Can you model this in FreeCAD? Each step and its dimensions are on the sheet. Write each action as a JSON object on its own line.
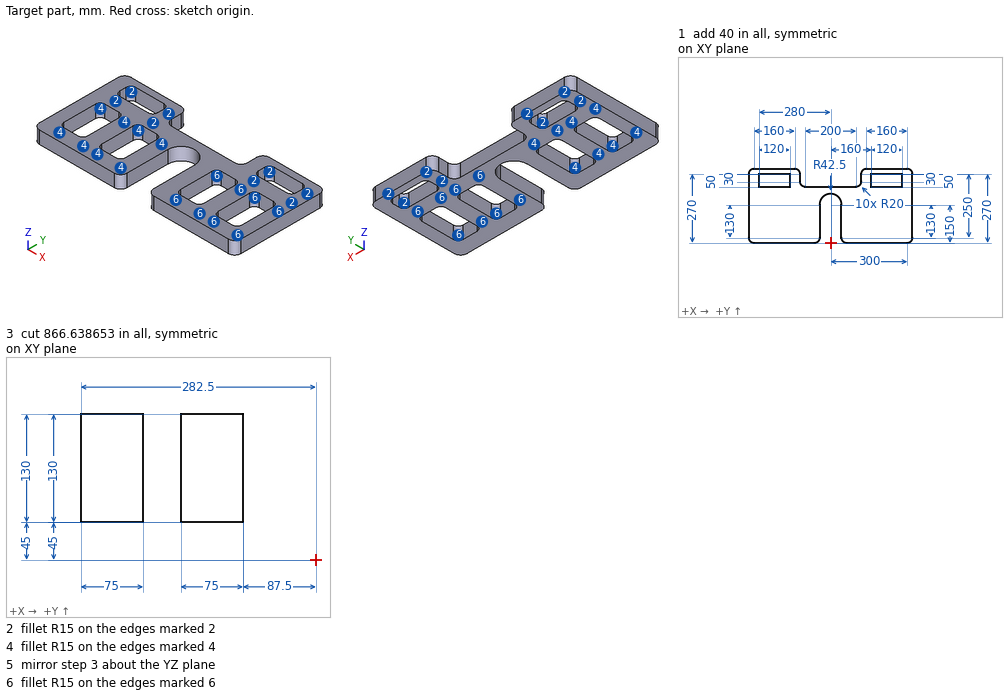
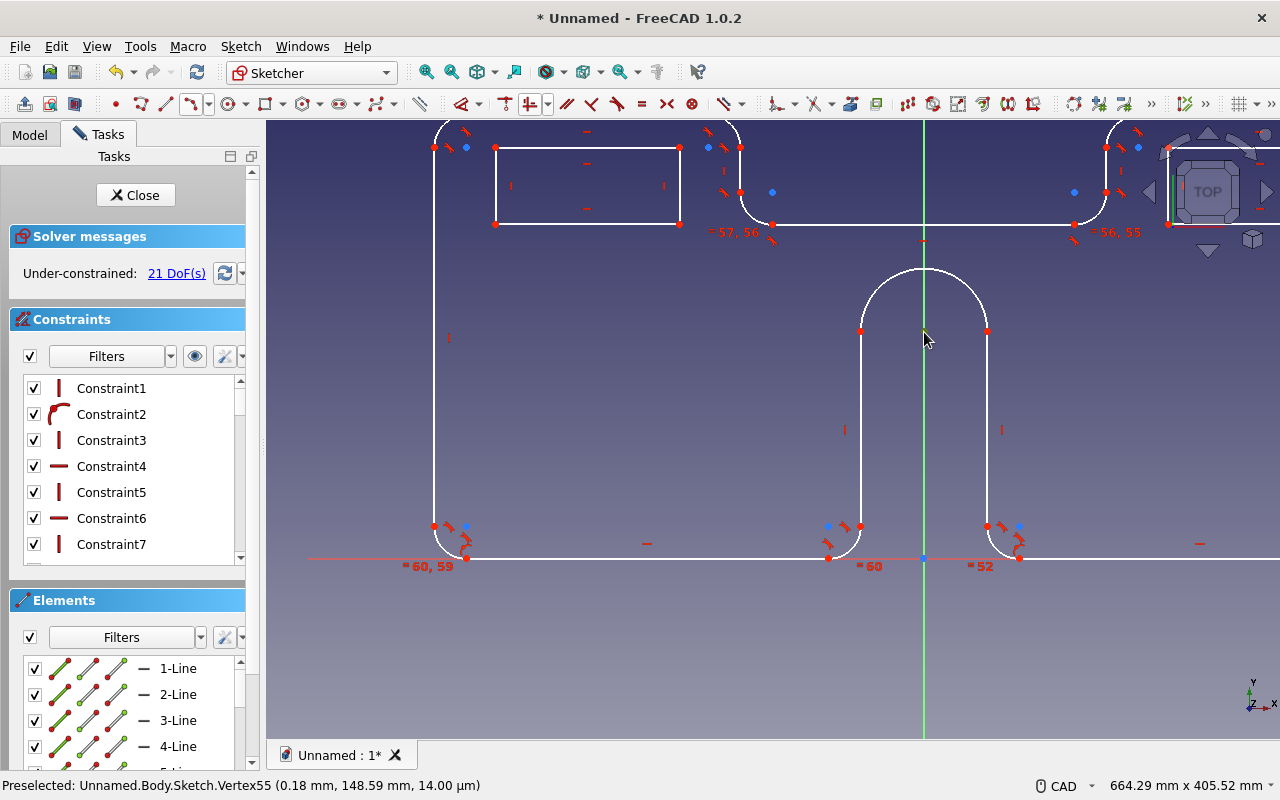
{"action": "left_click", "coordinate": [924, 671]}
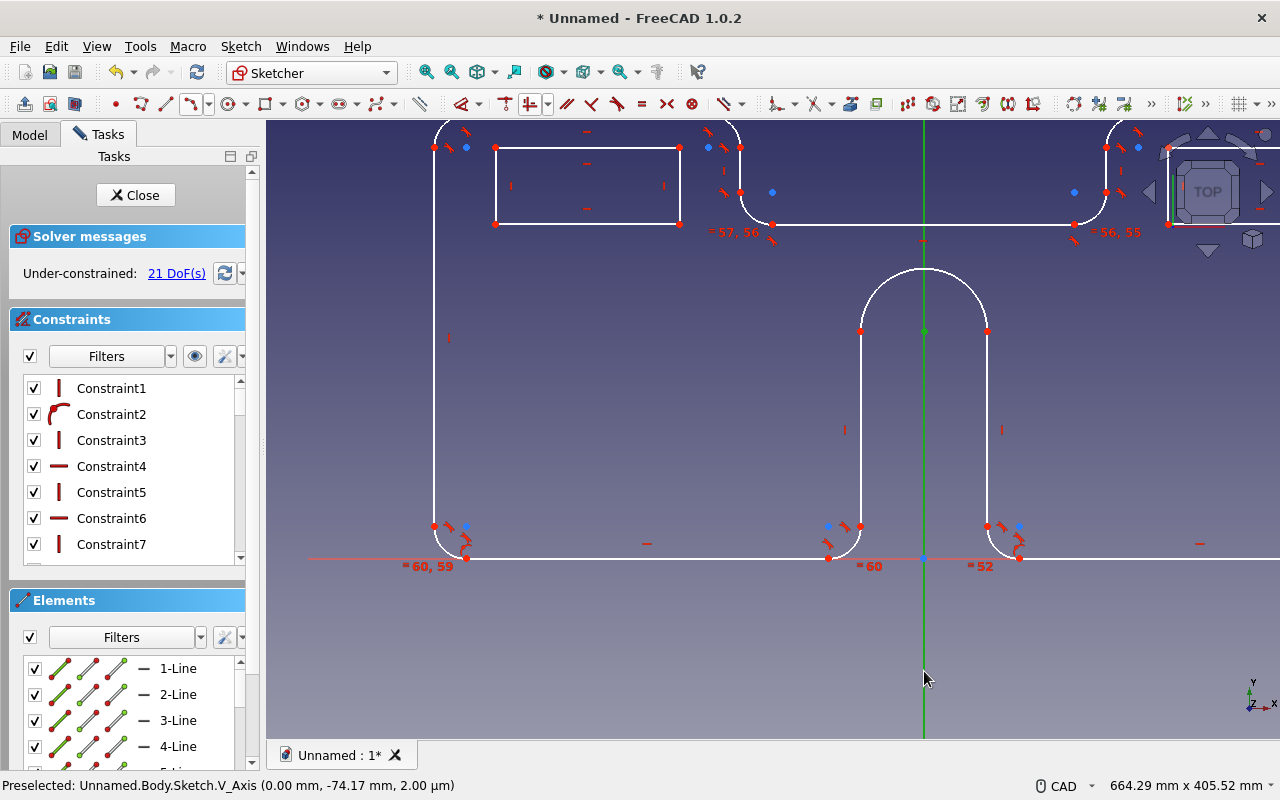
{"action": "key", "text": "c"}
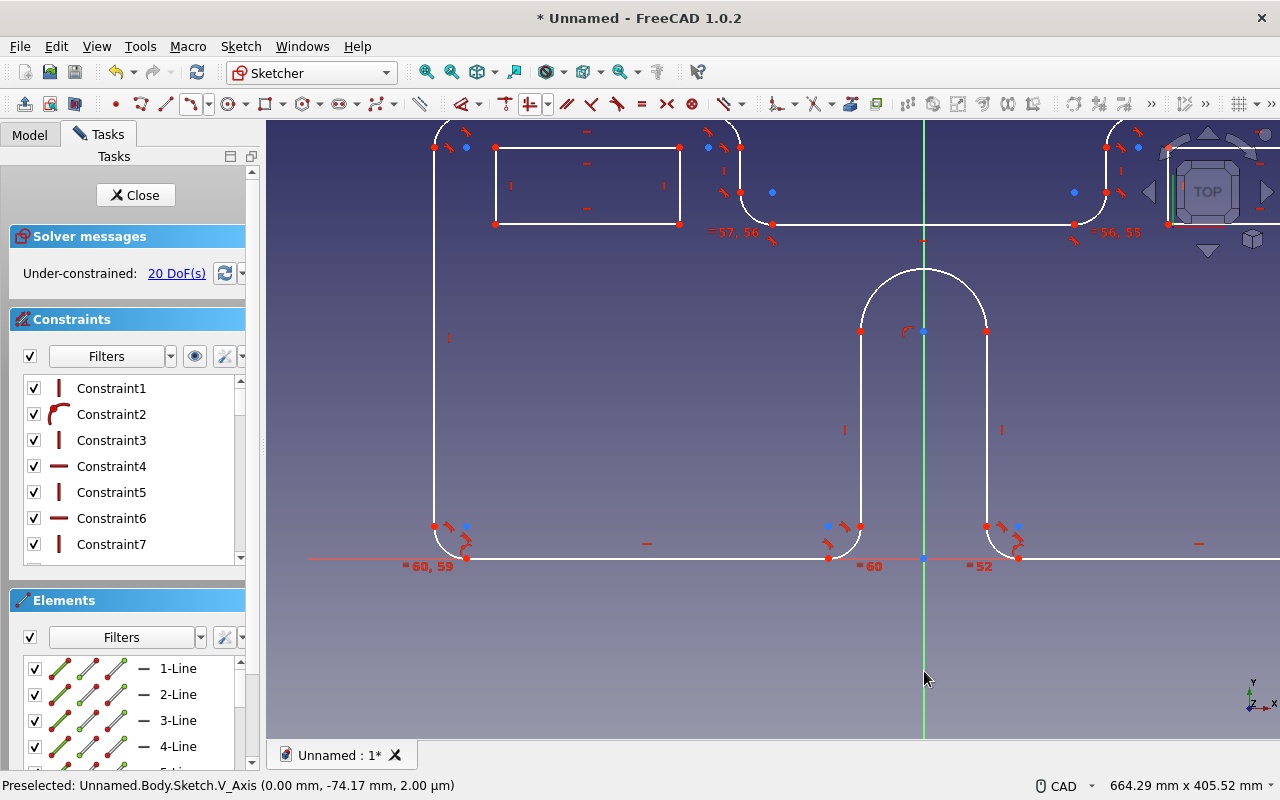
{"action": "key", "text": "d"}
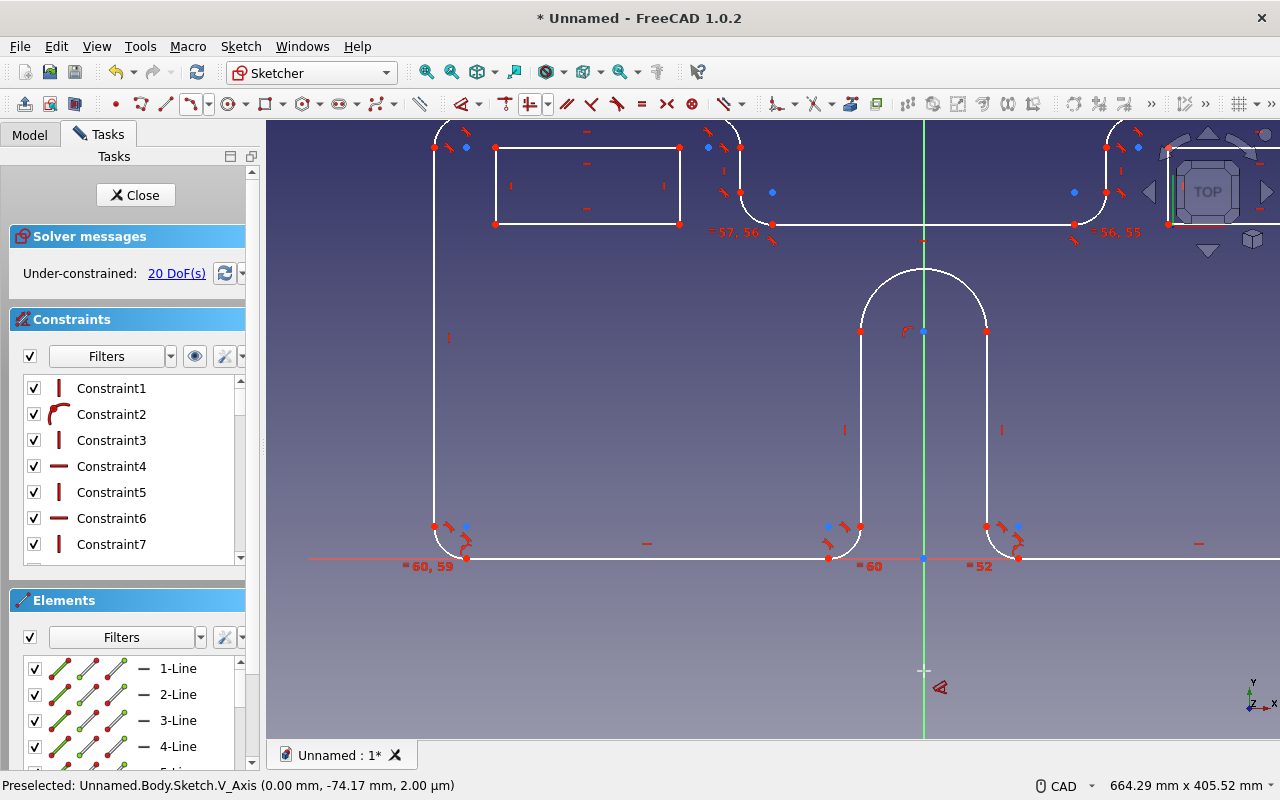
{"action": "scroll", "coordinate": [990, 541], "scroll_direction": "up", "scroll_amount": 2}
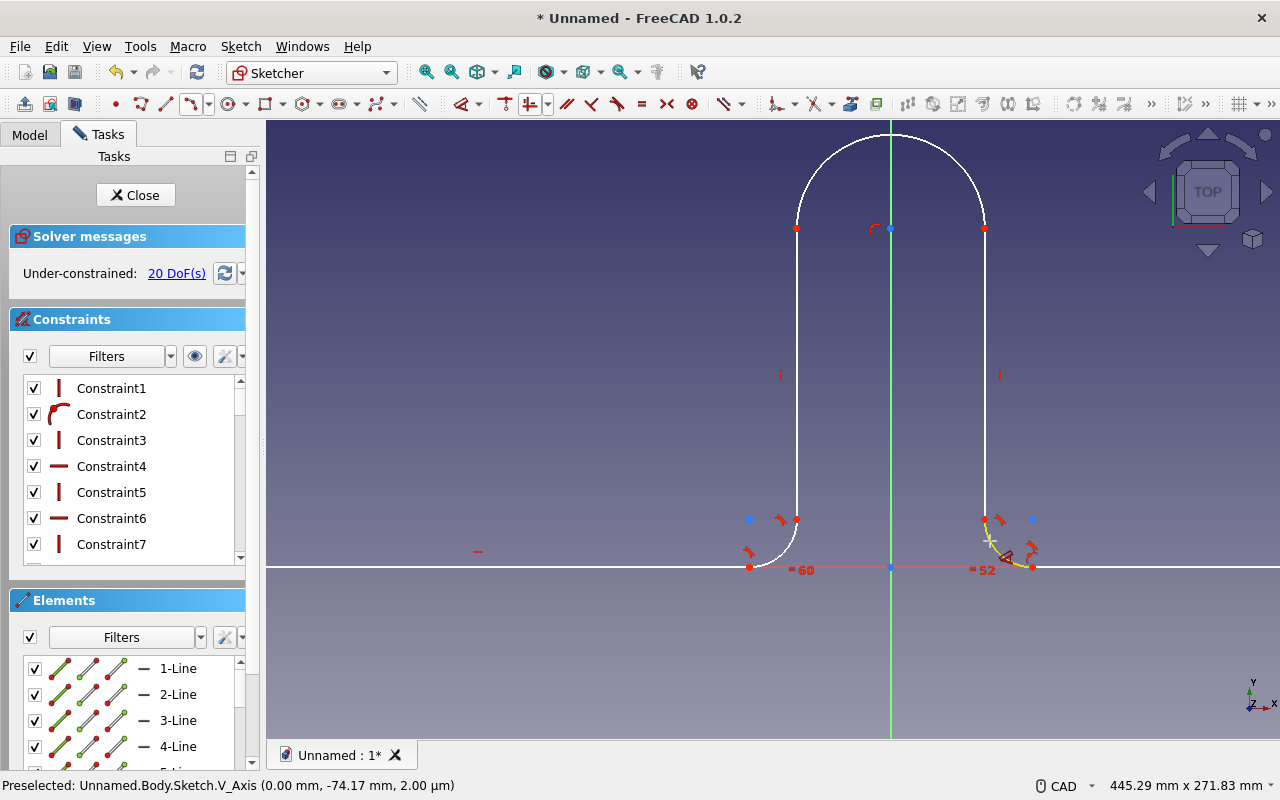
{"action": "left_click", "coordinate": [990, 541]}
{"action": "left_click", "coordinate": [953, 517]}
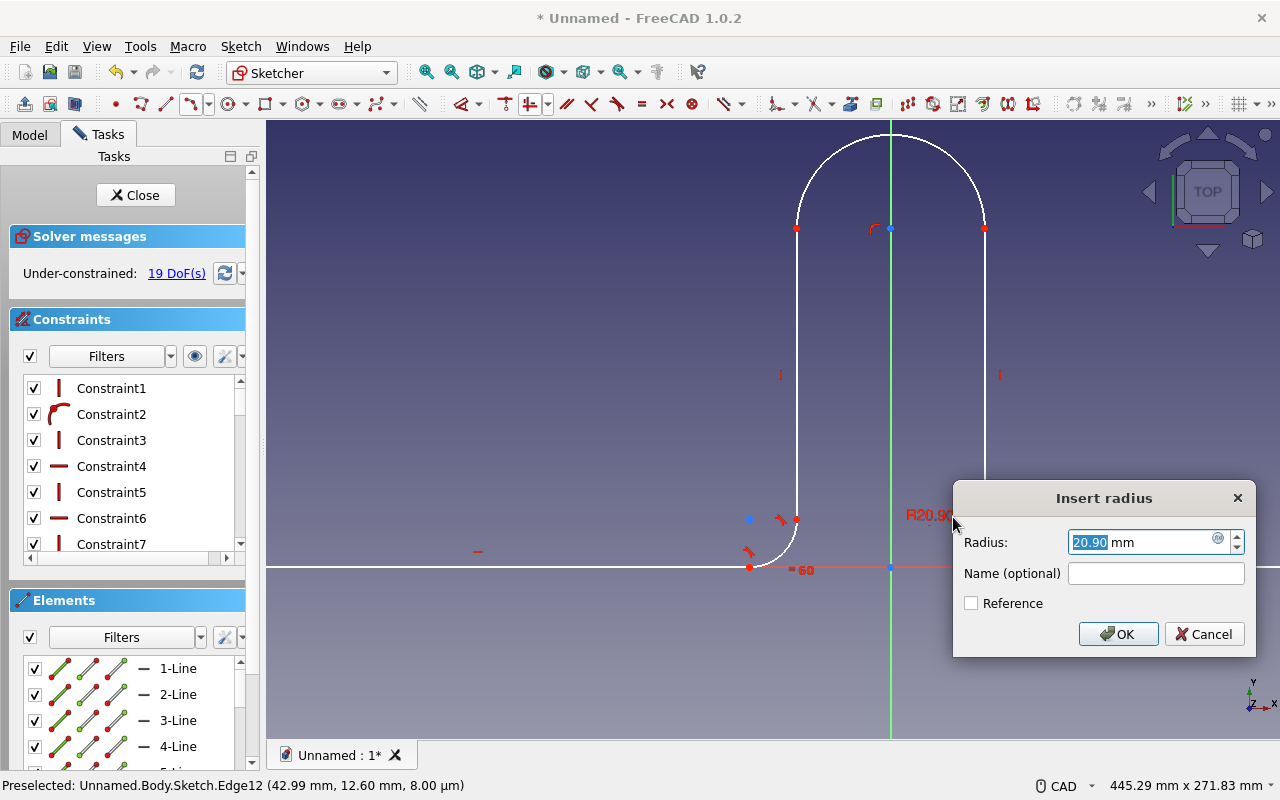
{"action": "type", "text": "20"}
{"action": "key", "text": "Return"}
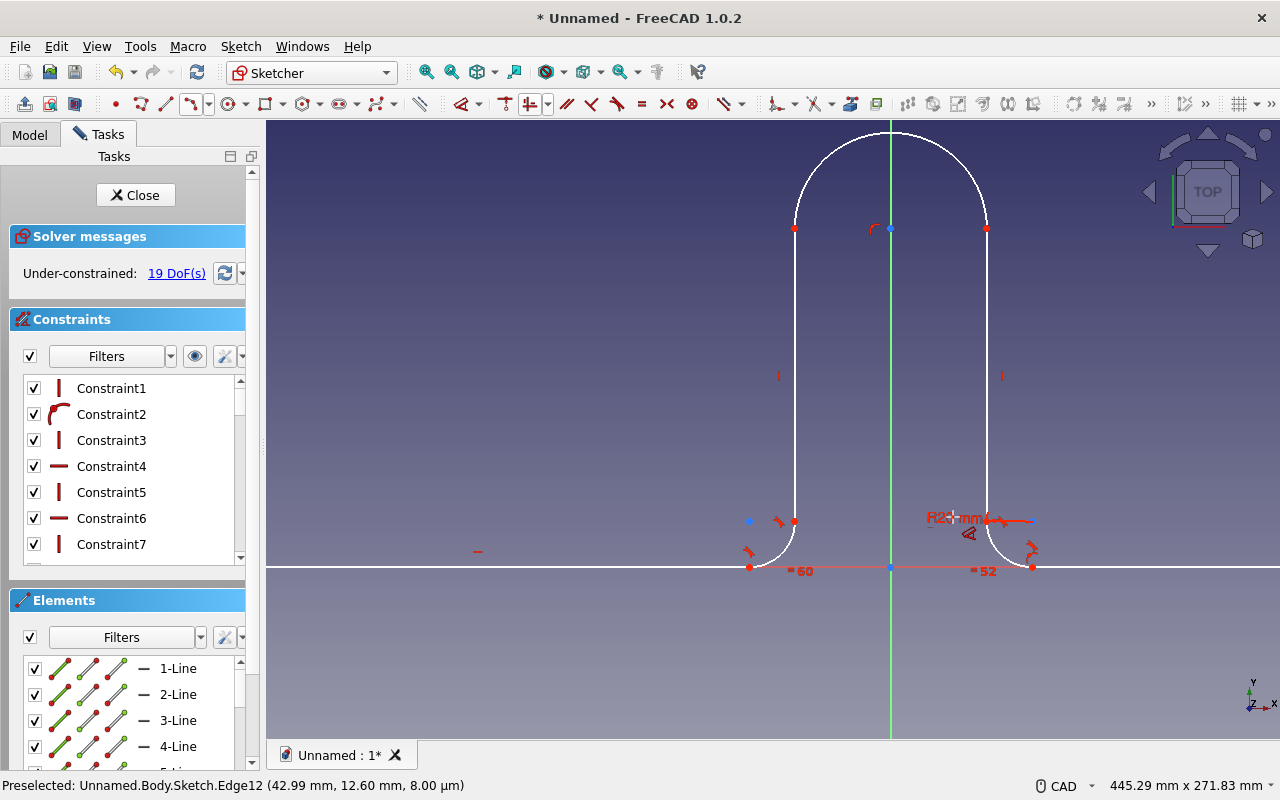
{"action": "left_click", "coordinate": [947, 151]}
{"action": "left_click", "coordinate": [1006, 174]}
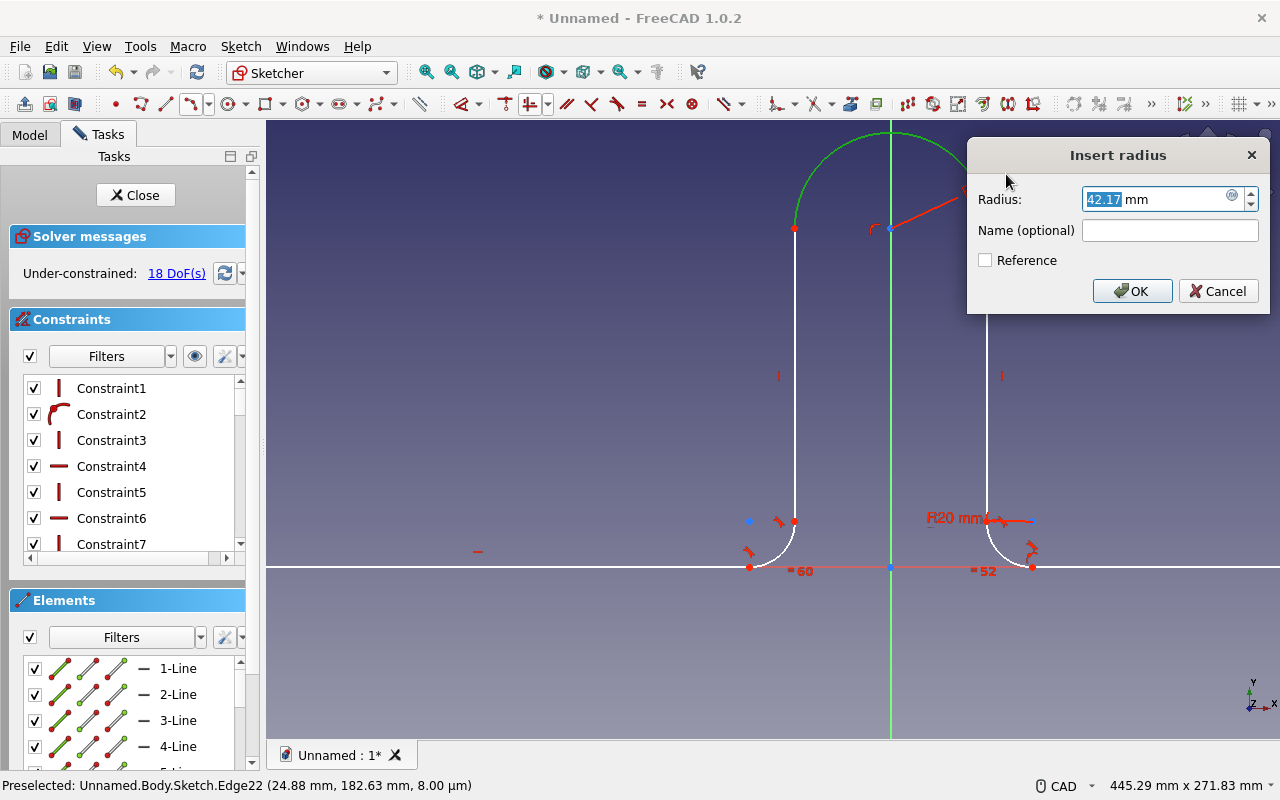
{"action": "type", "text": "42.5"}
{"action": "key", "text": "Return"}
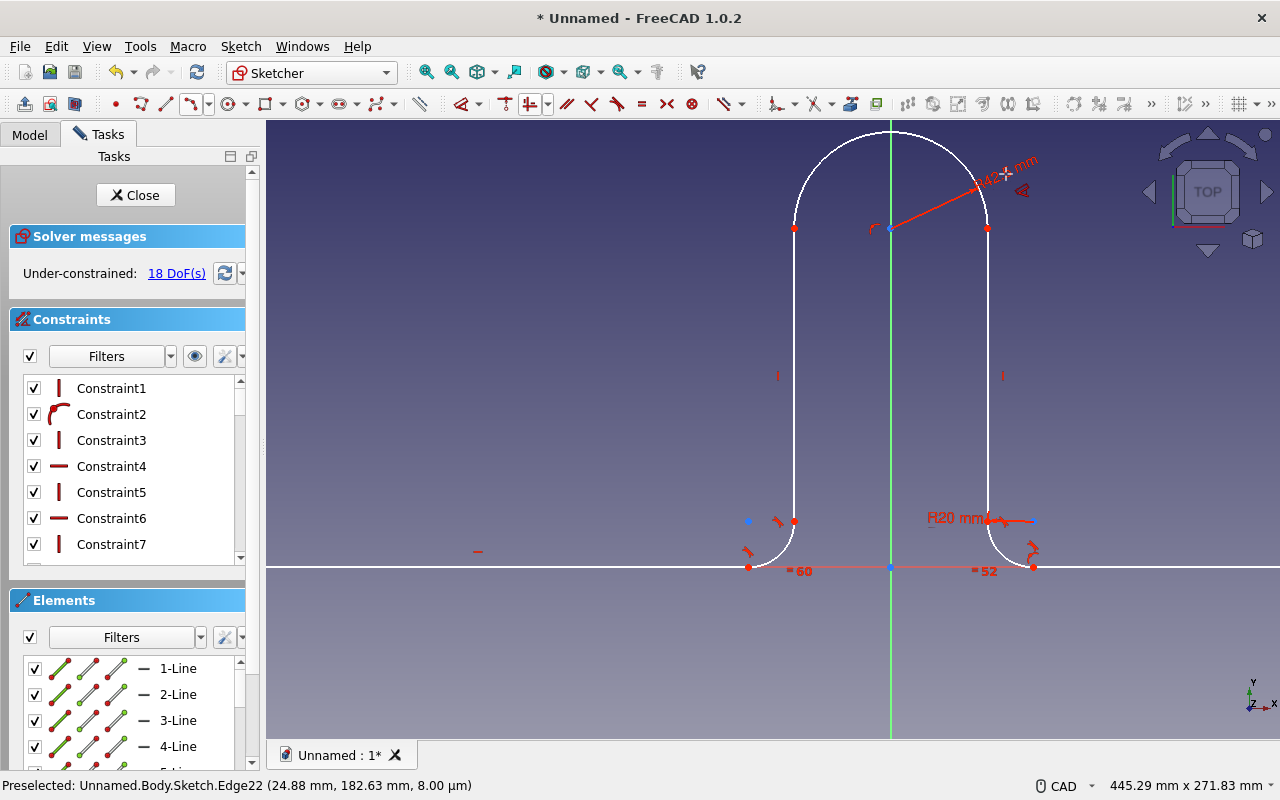
{"action": "scroll", "coordinate": [596, 542], "scroll_direction": "down", "scroll_amount": 5}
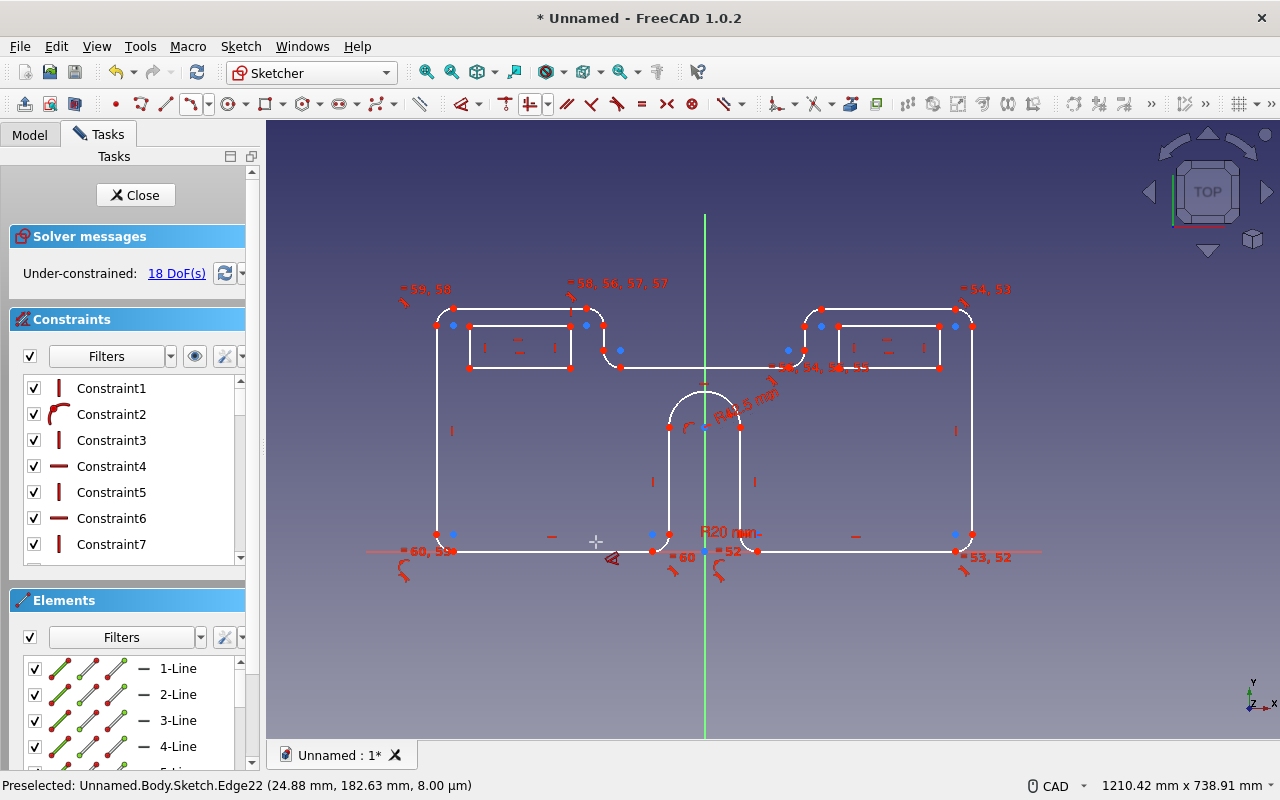
{"action": "scroll", "coordinate": [805, 334], "scroll_direction": "up", "scroll_amount": 4}